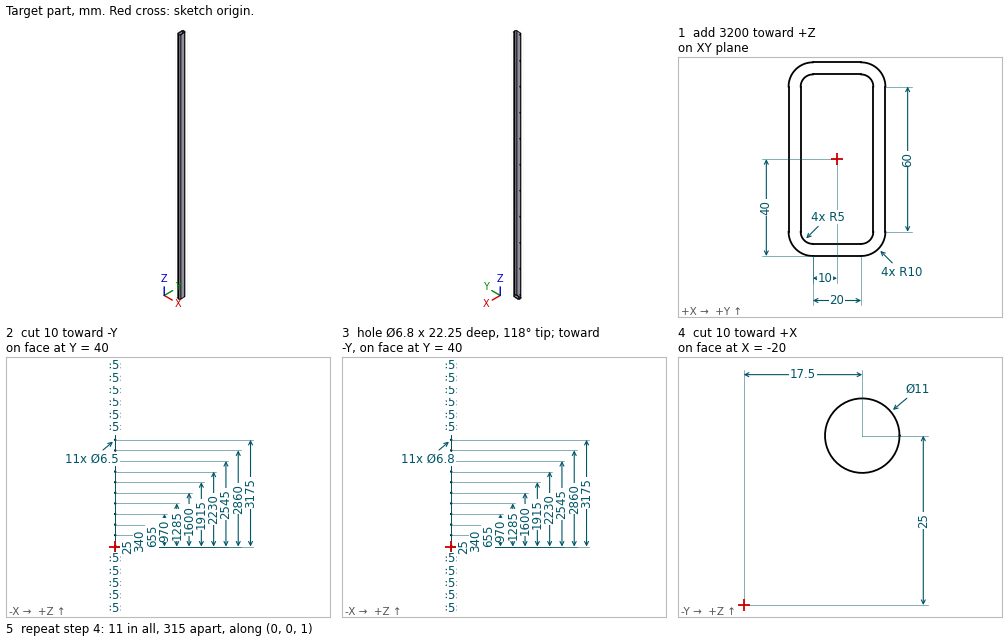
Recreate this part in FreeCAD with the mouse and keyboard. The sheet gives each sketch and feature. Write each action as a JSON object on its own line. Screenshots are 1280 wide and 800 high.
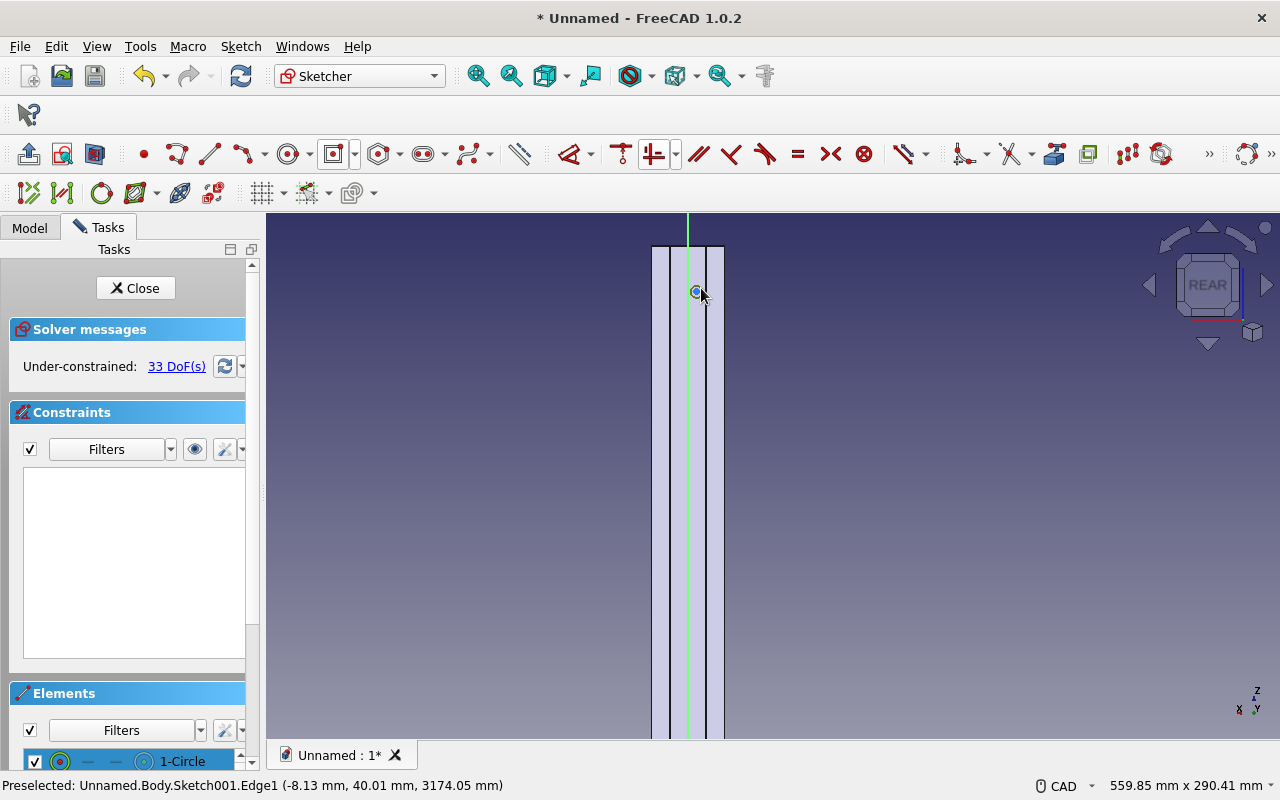
{"action": "scroll", "coordinate": [705, 302], "scroll_direction": "down", "scroll_amount": 14}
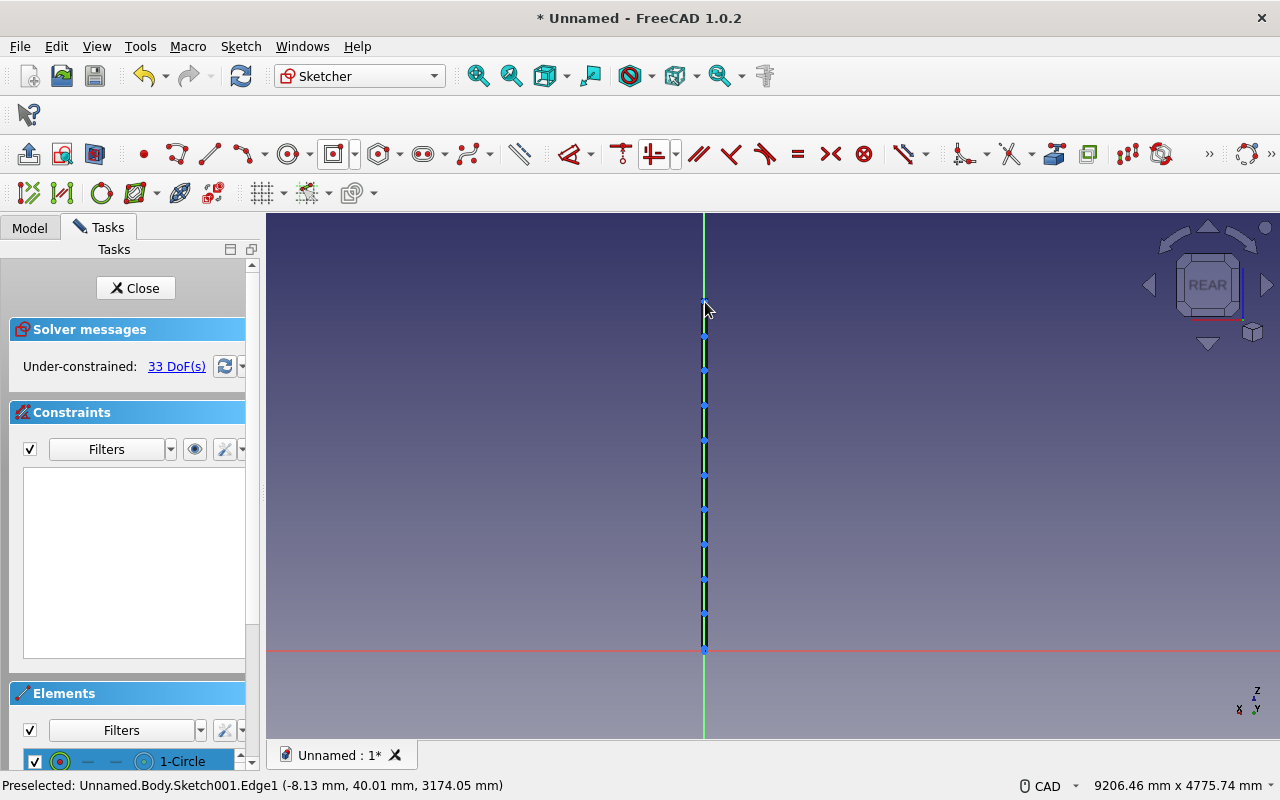
{"action": "scroll", "coordinate": [705, 336], "scroll_direction": "up", "scroll_amount": 14}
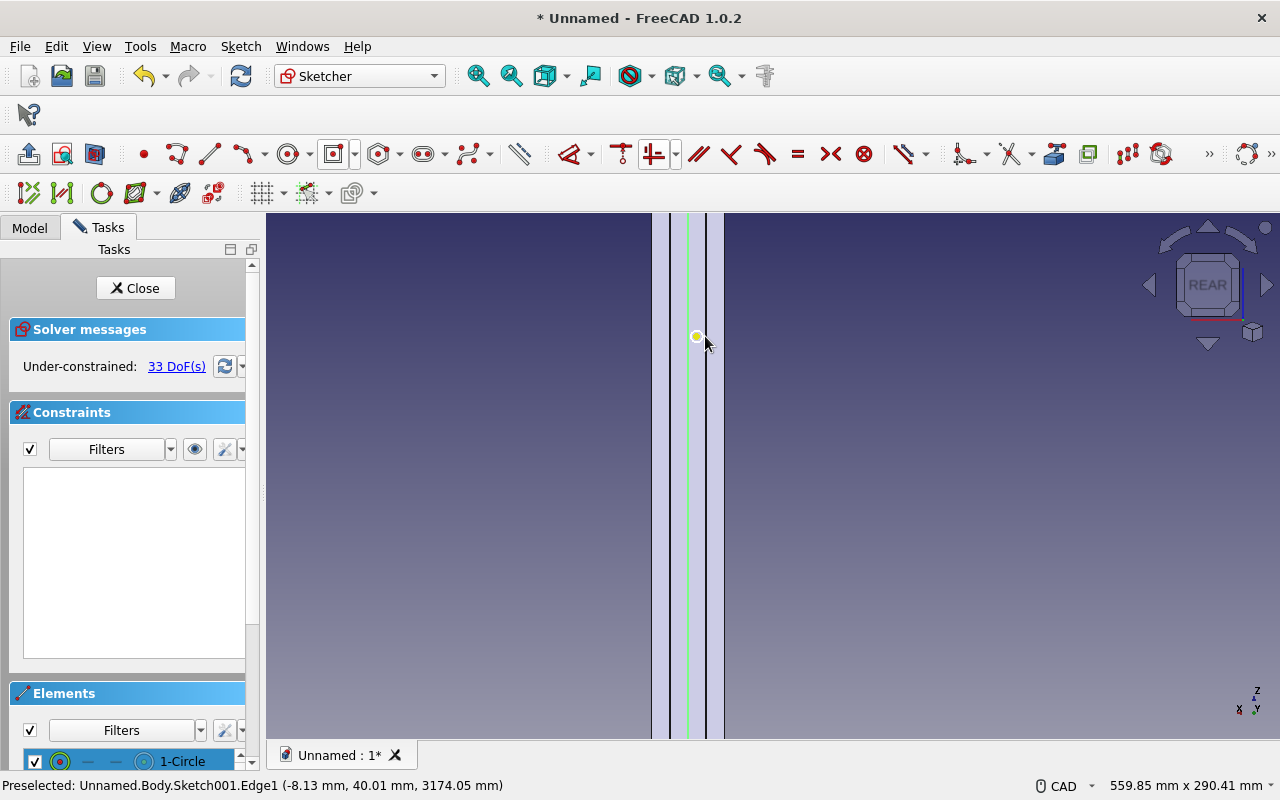
{"action": "left_click", "coordinate": [701, 332]}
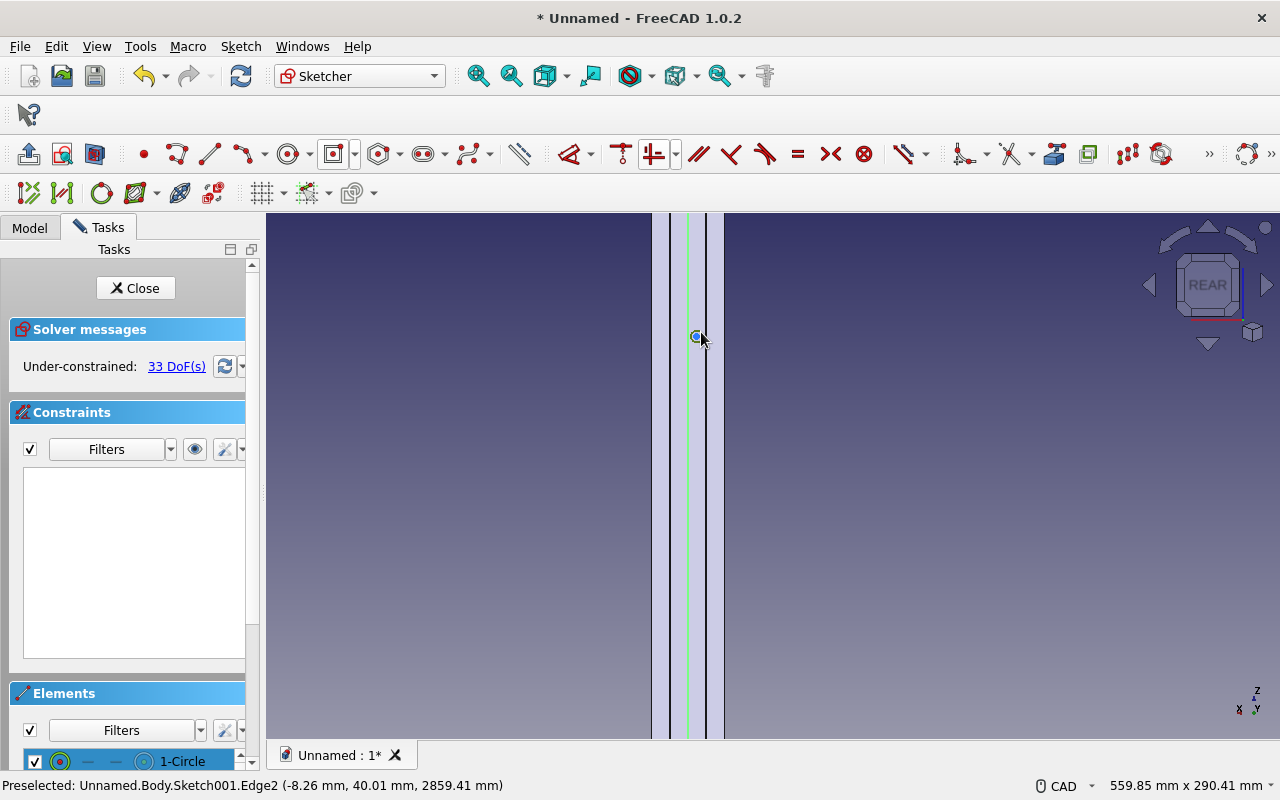
{"action": "scroll", "coordinate": [705, 336], "scroll_direction": "down", "scroll_amount": 14}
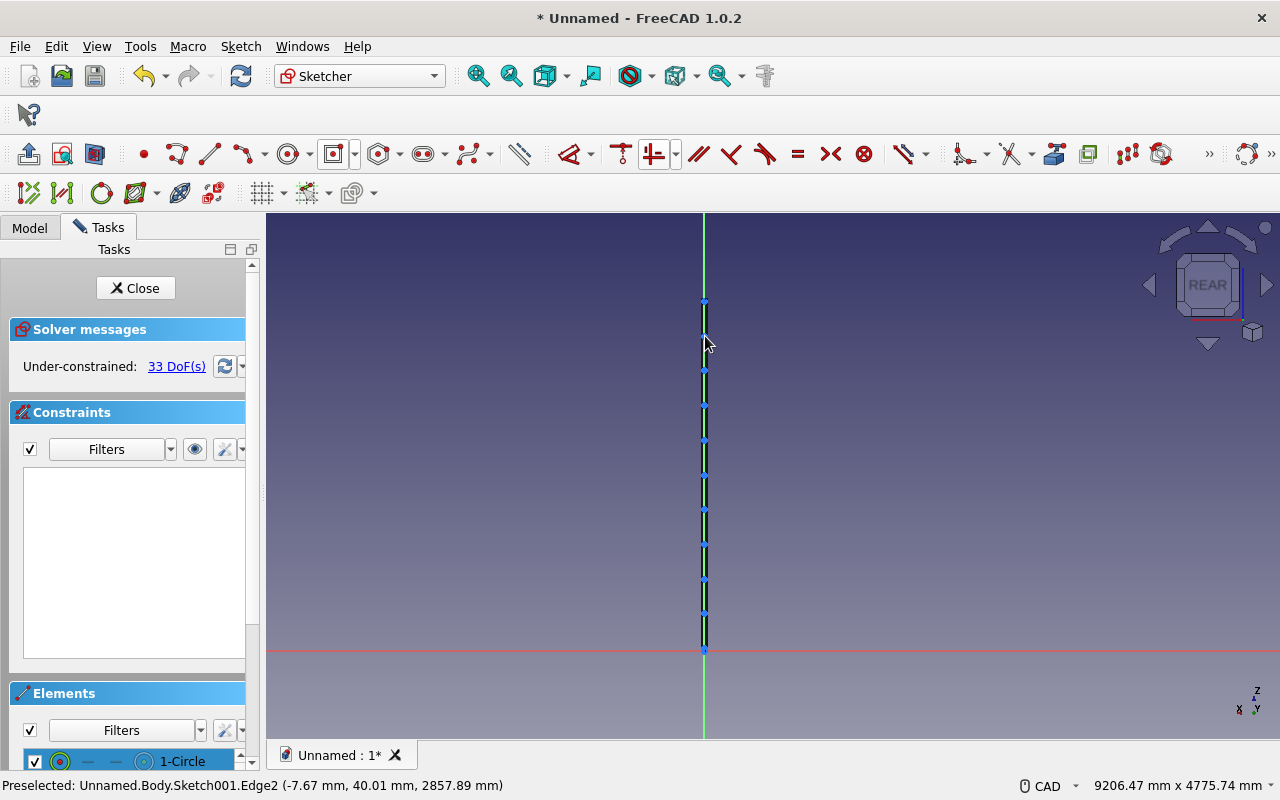
{"action": "scroll", "coordinate": [705, 371], "scroll_direction": "up", "scroll_amount": 14}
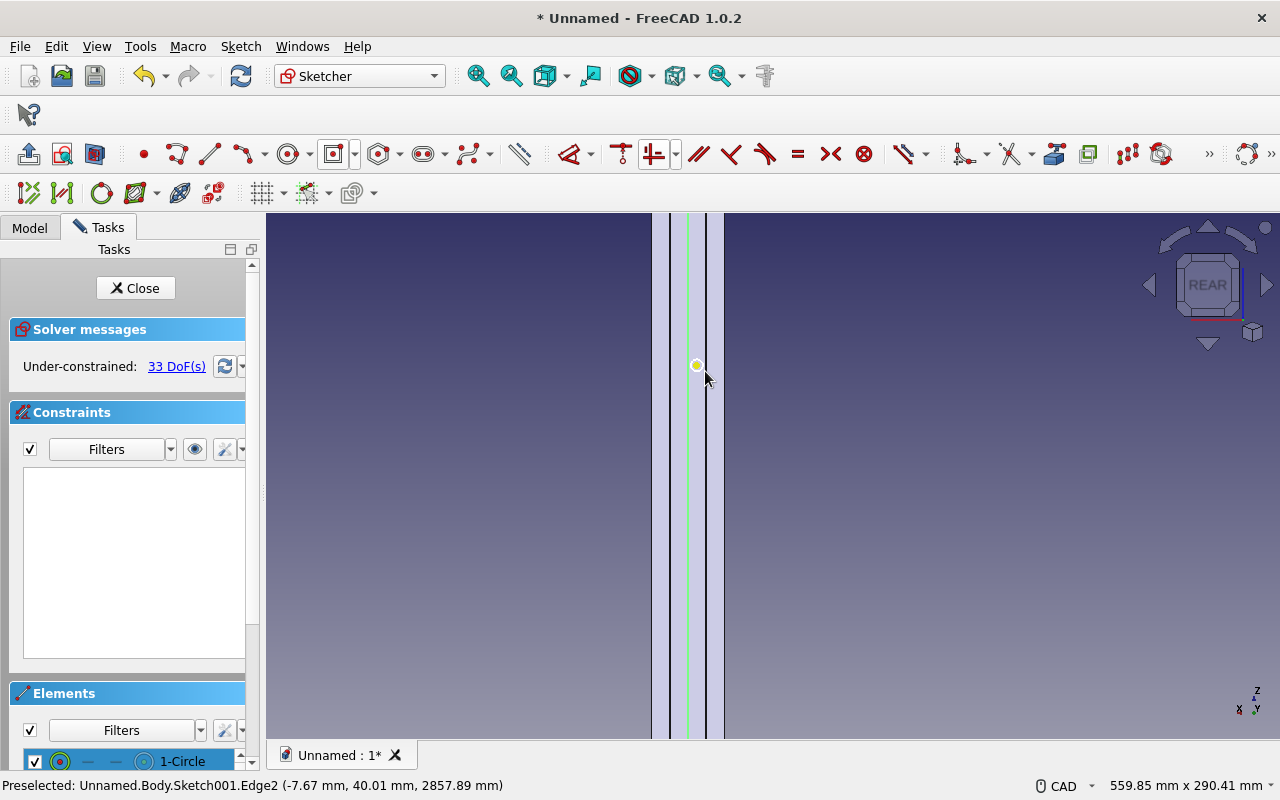
{"action": "left_click", "coordinate": [701, 370]}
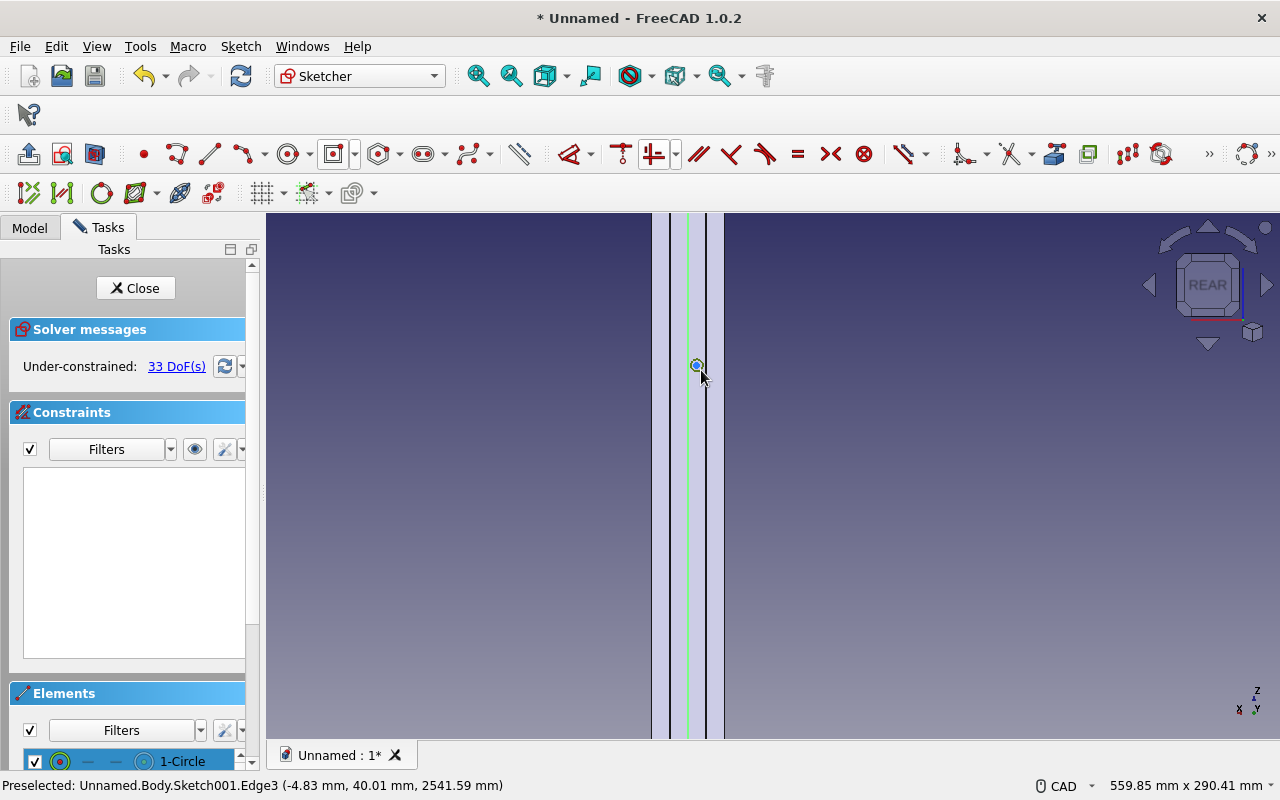
{"action": "scroll", "coordinate": [705, 371], "scroll_direction": "down", "scroll_amount": 14}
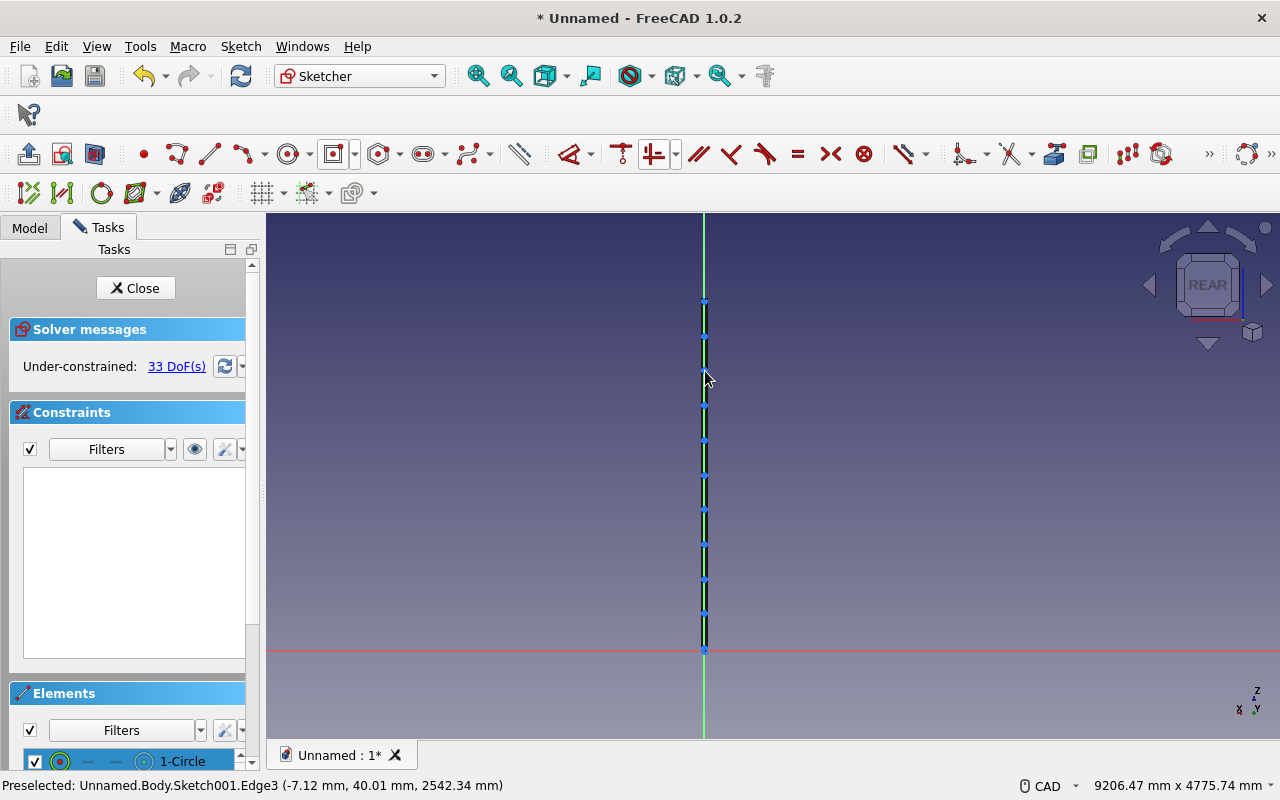
{"action": "scroll", "coordinate": [705, 406], "scroll_direction": "up", "scroll_amount": 14}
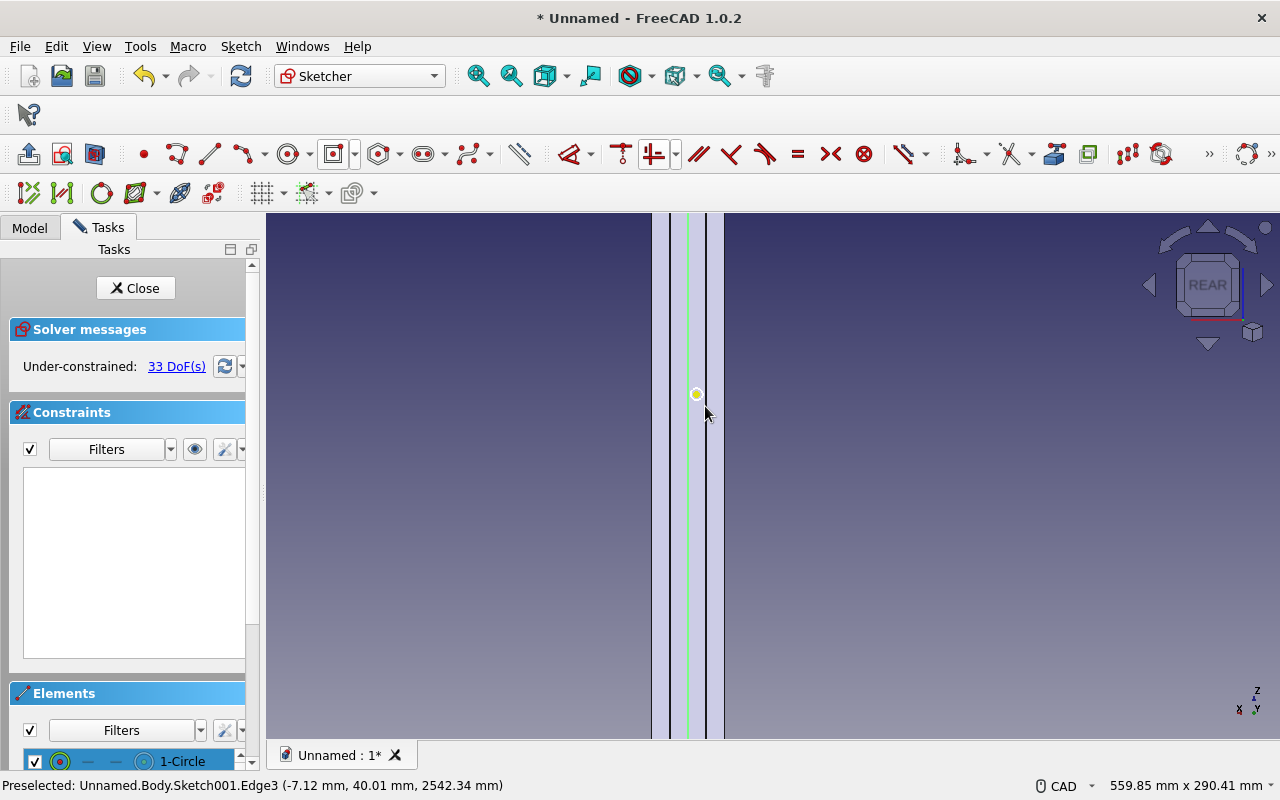
{"action": "left_click", "coordinate": [701, 398]}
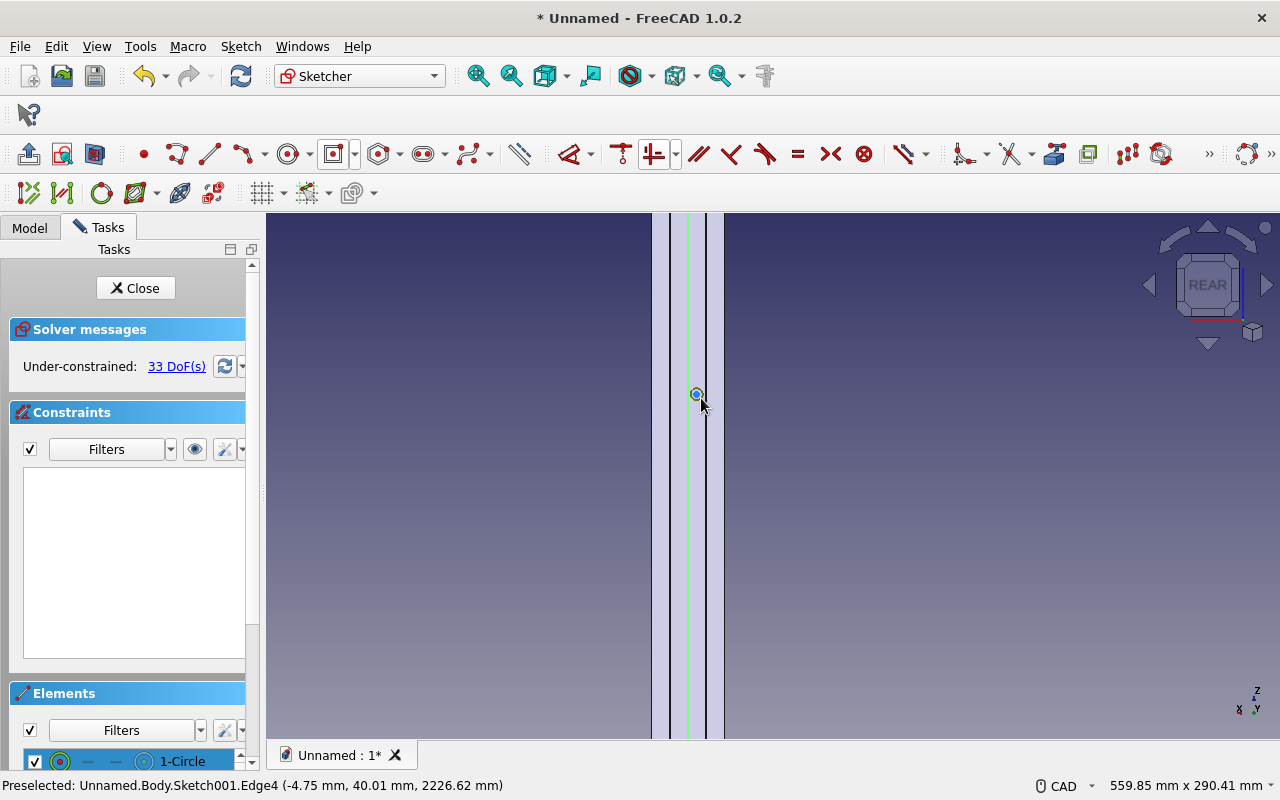
{"action": "scroll", "coordinate": [705, 406], "scroll_direction": "down", "scroll_amount": 14}